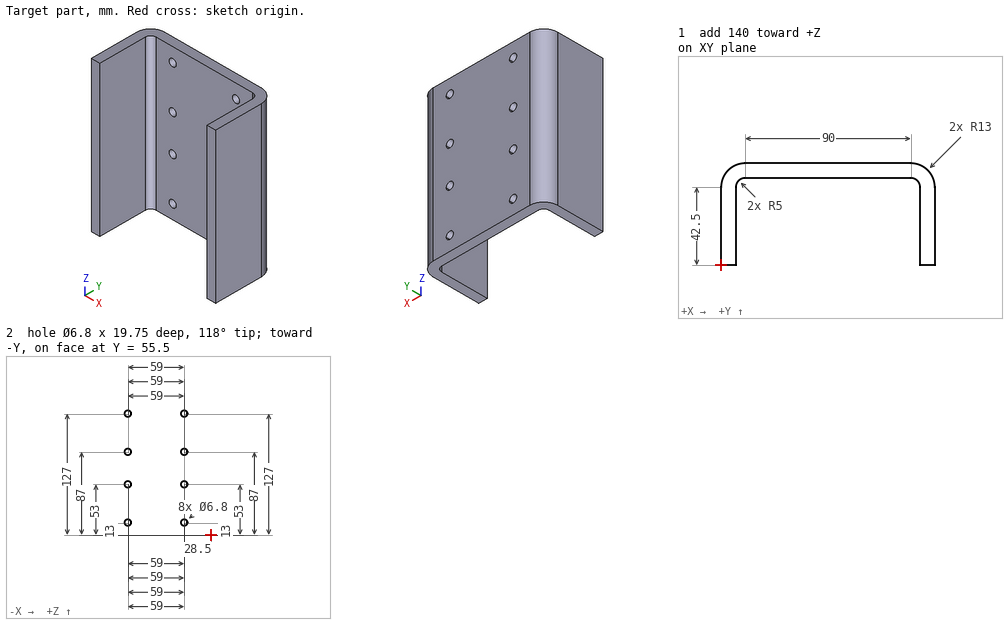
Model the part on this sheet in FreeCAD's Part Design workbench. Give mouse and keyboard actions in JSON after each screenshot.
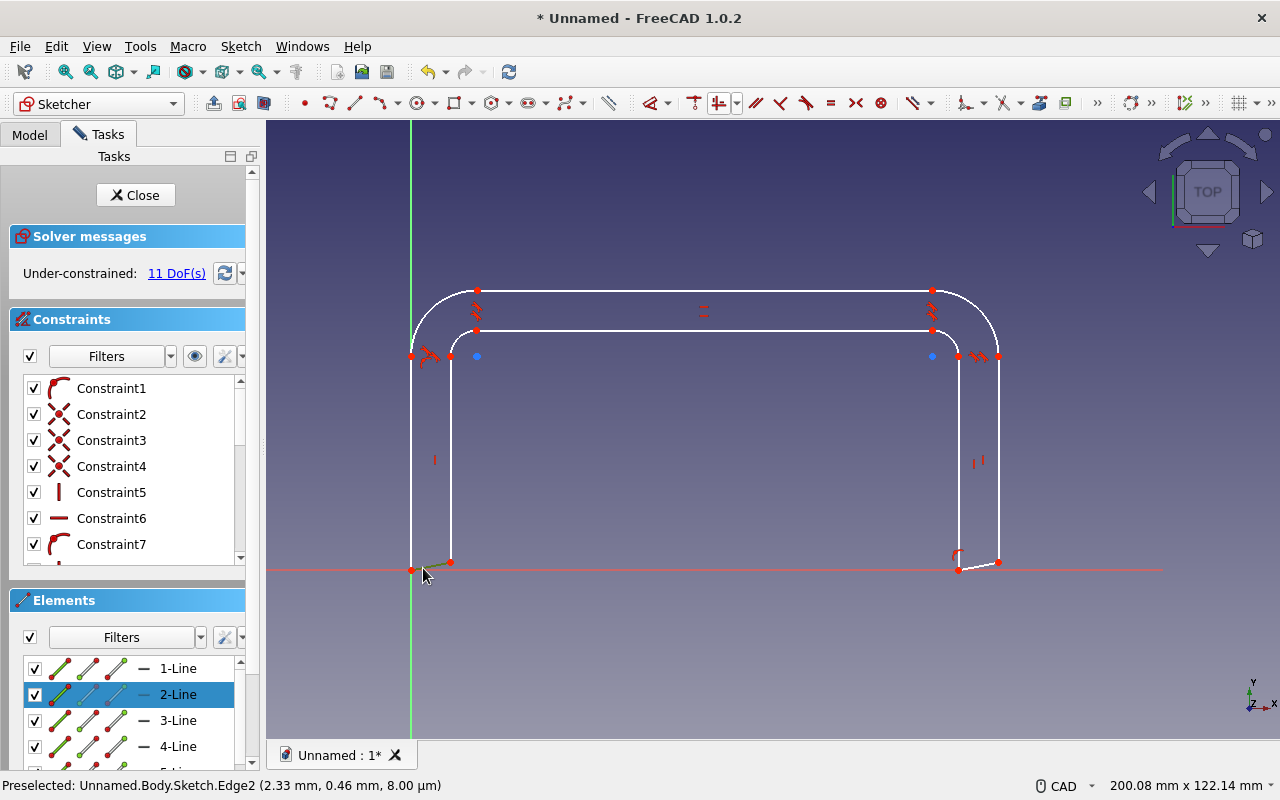
{"action": "key", "text": "h"}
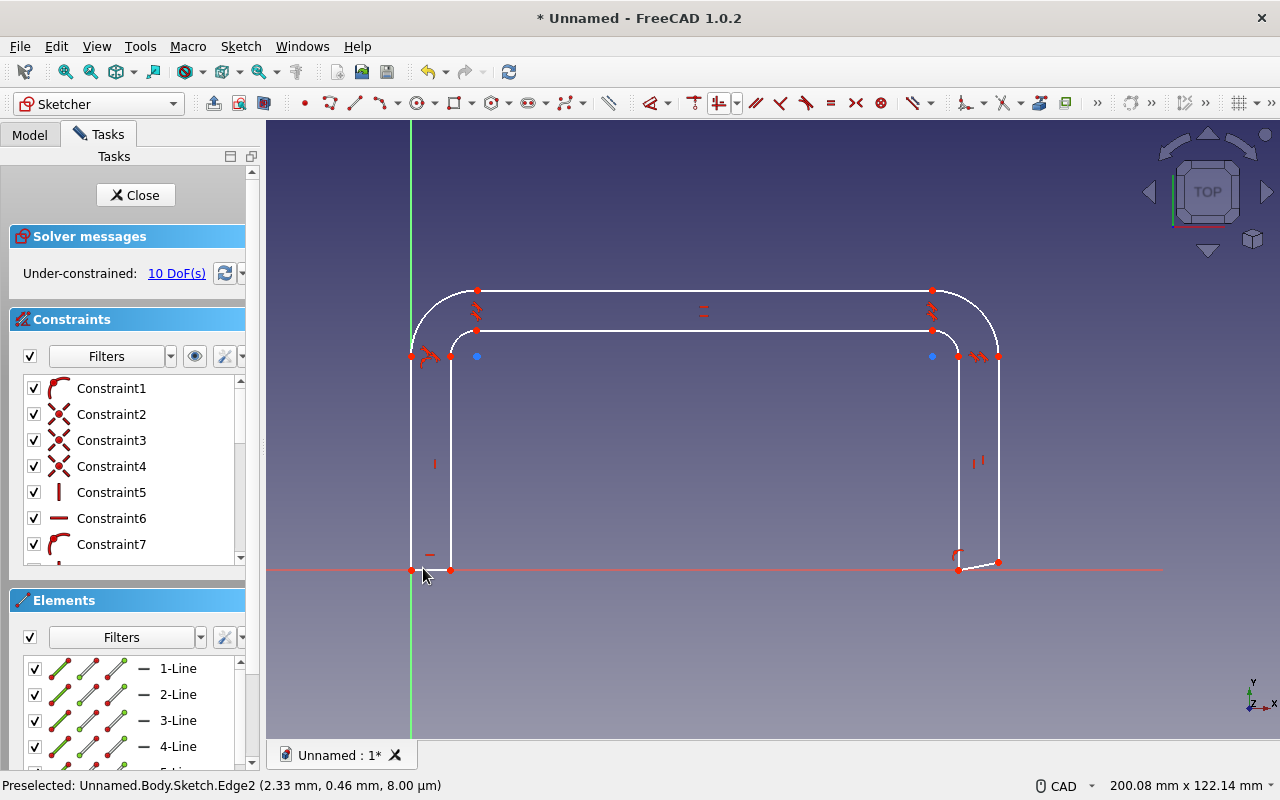
{"action": "left_click", "coordinate": [971, 568]}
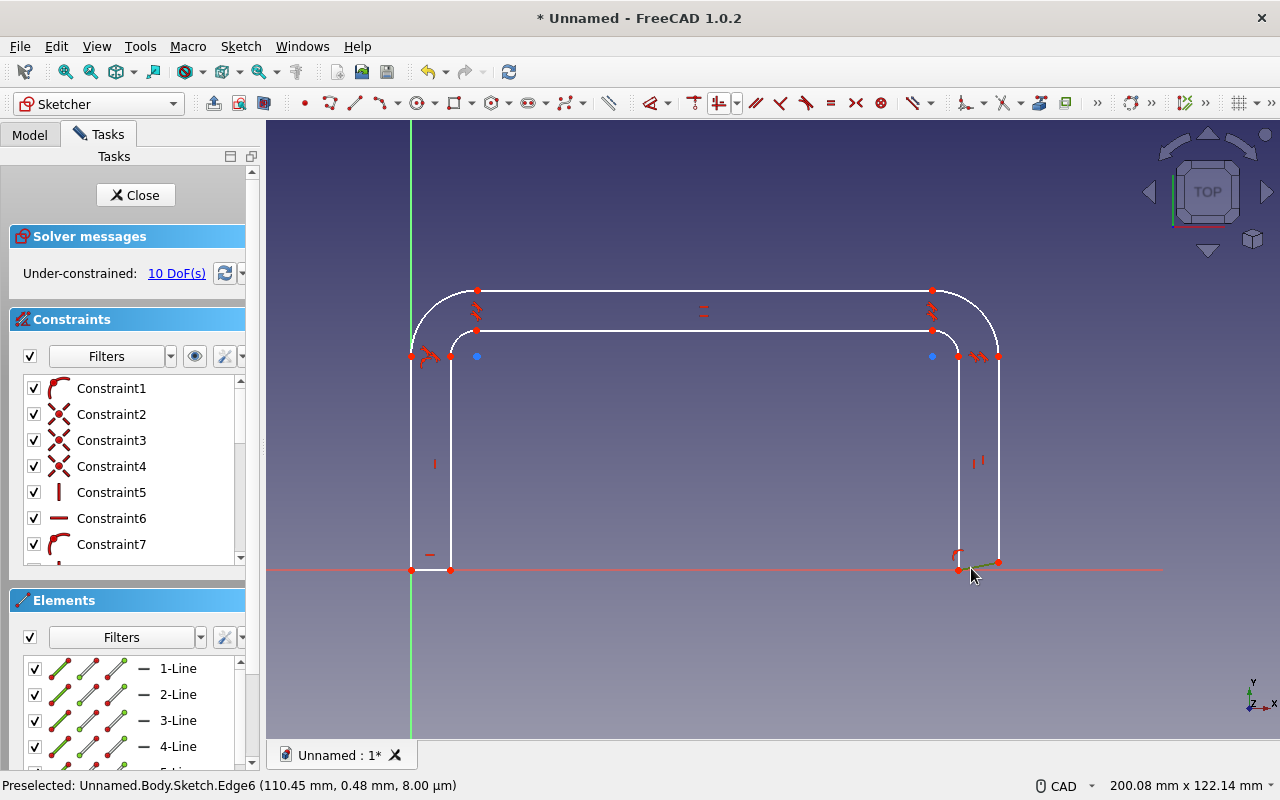
{"action": "left_click", "coordinate": [736, 104]}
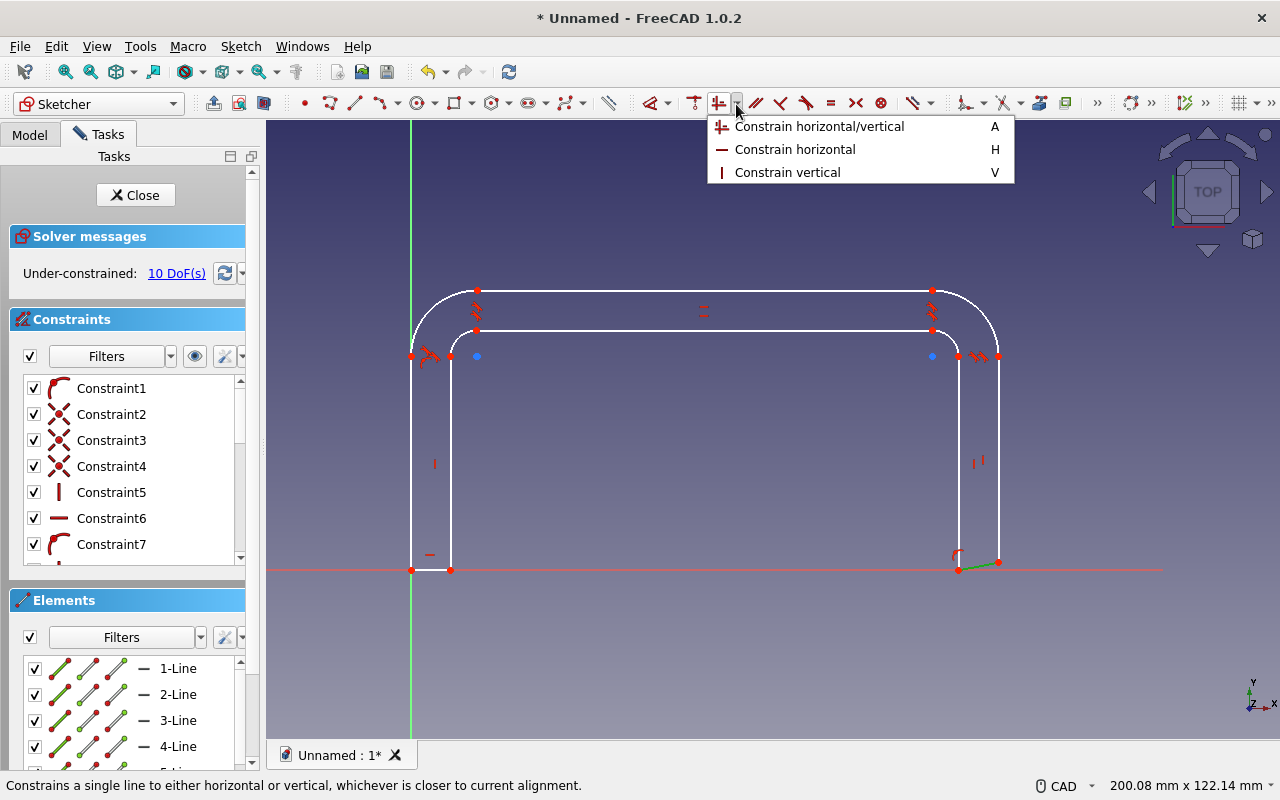
{"action": "left_click", "coordinate": [861, 150]}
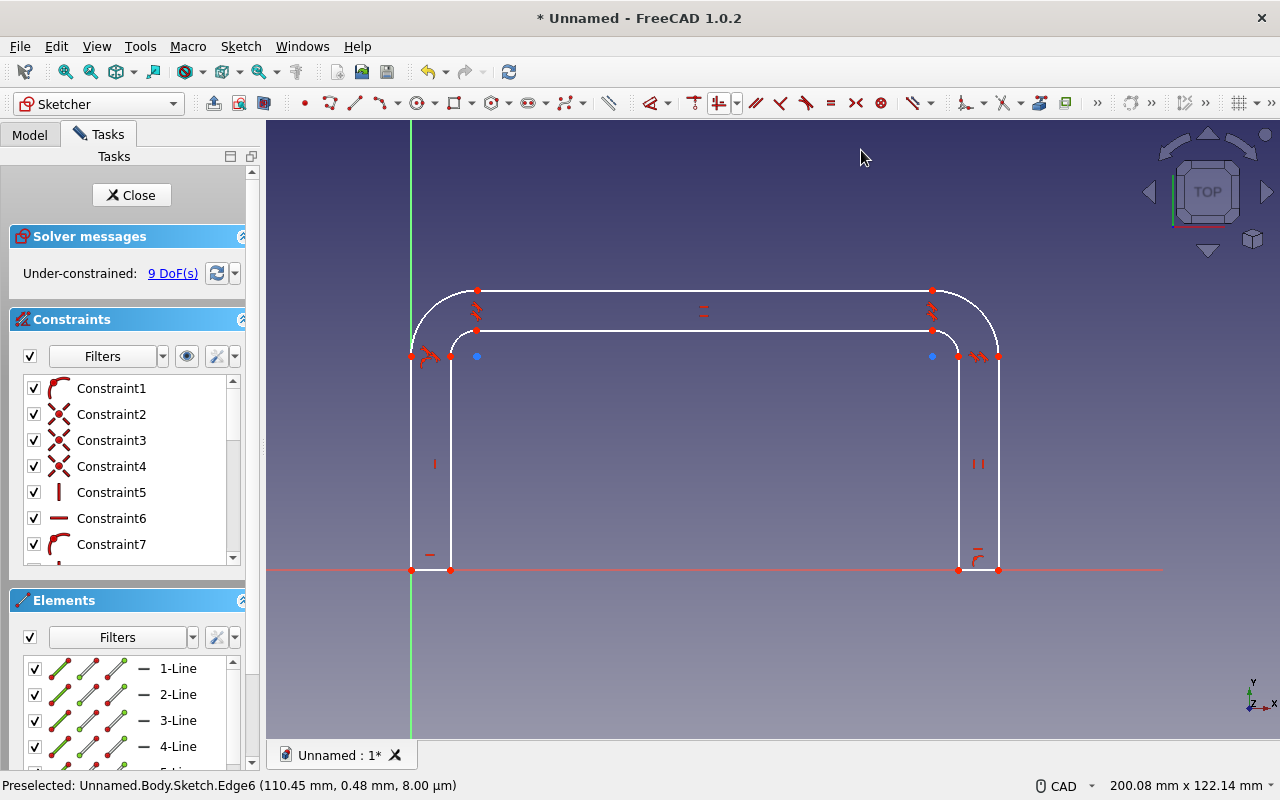
{"action": "left_click", "coordinate": [956, 345]}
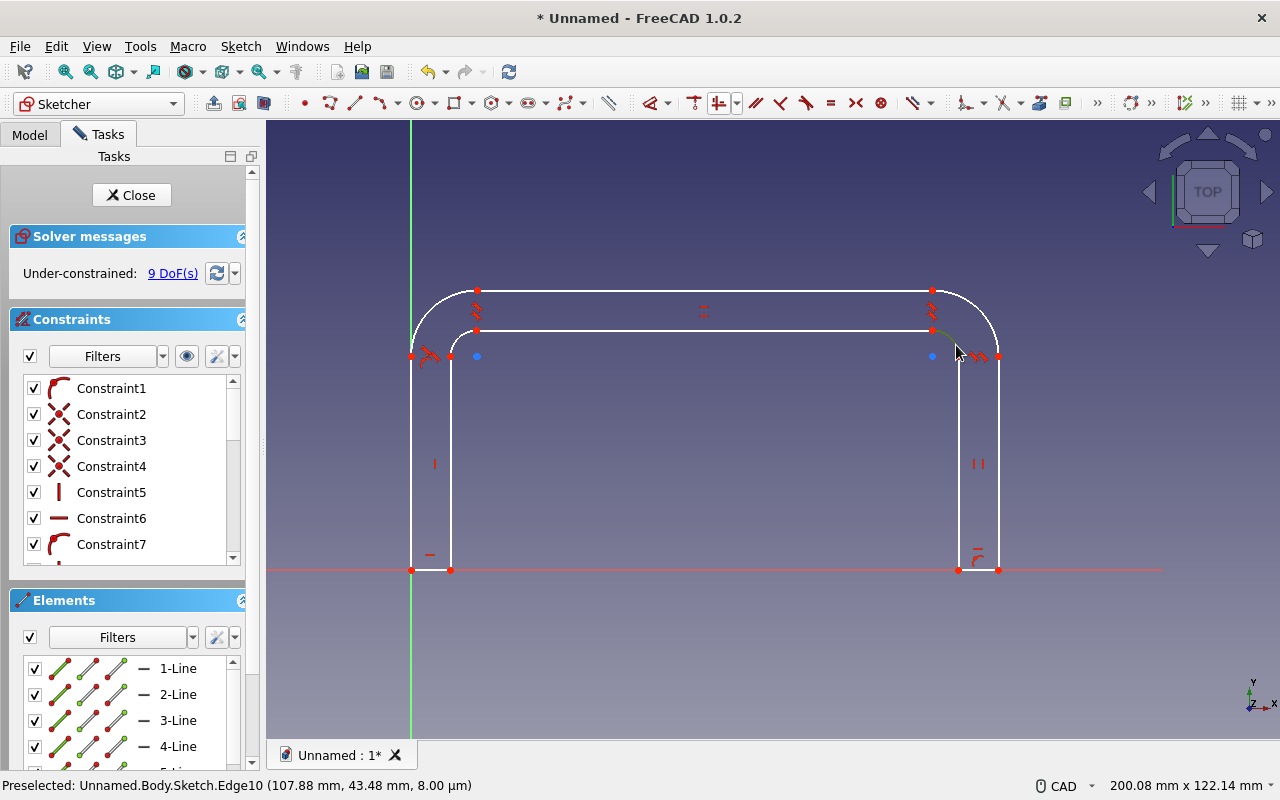
{"action": "left_click", "coordinate": [991, 327]}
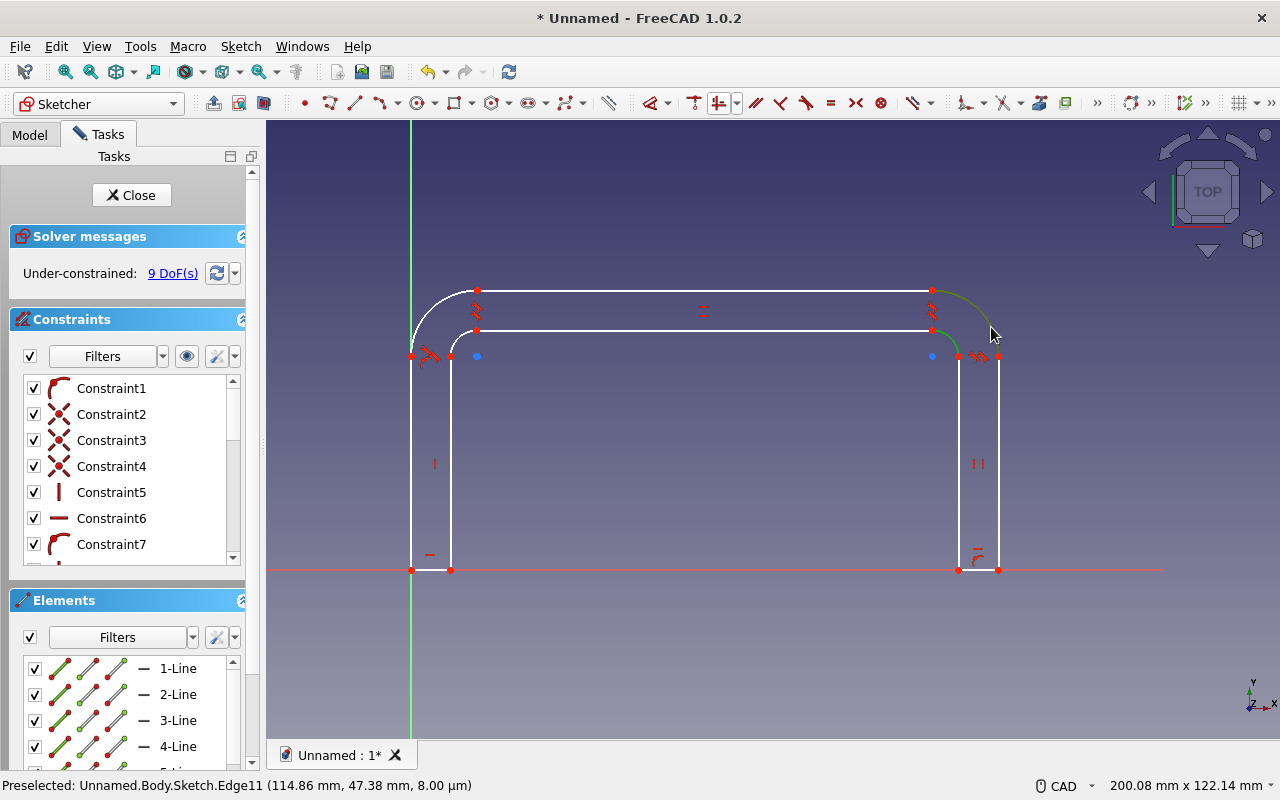
{"action": "key", "text": "c"}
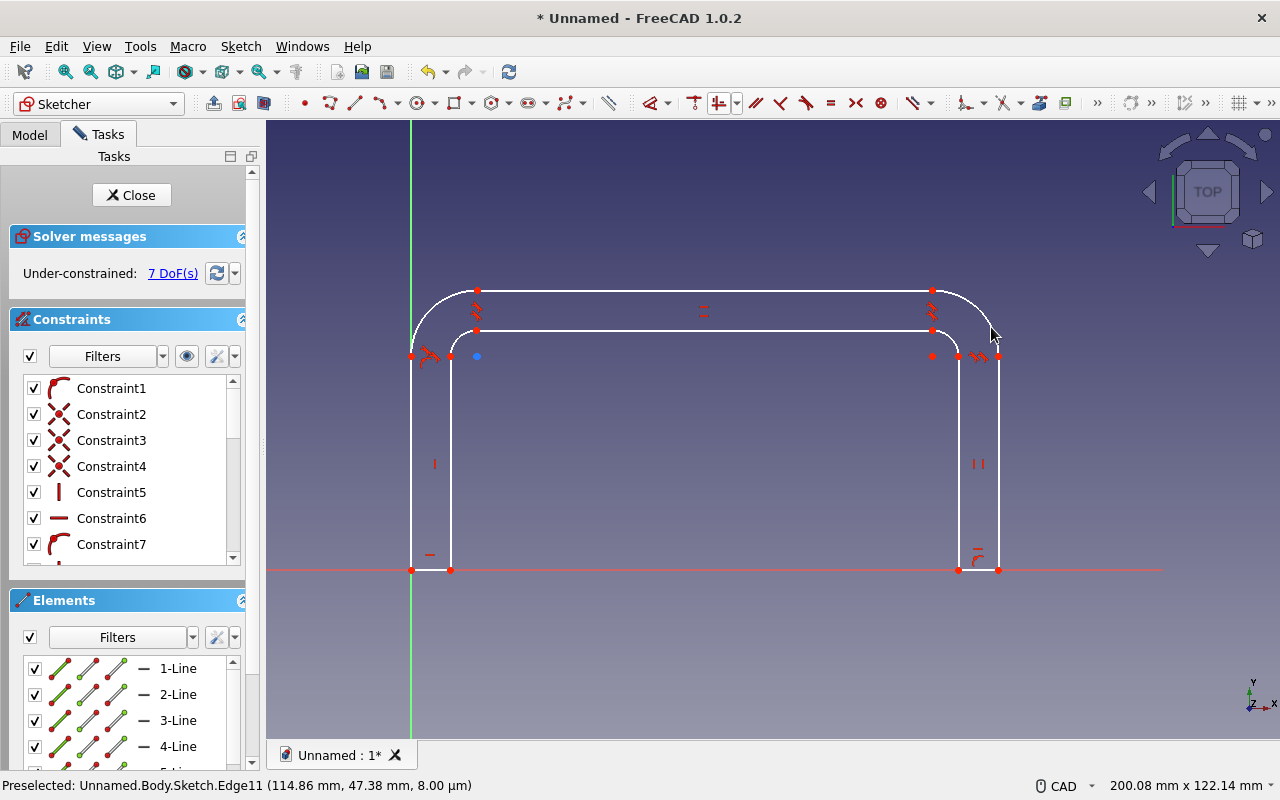
{"action": "left_click", "coordinate": [465, 333]}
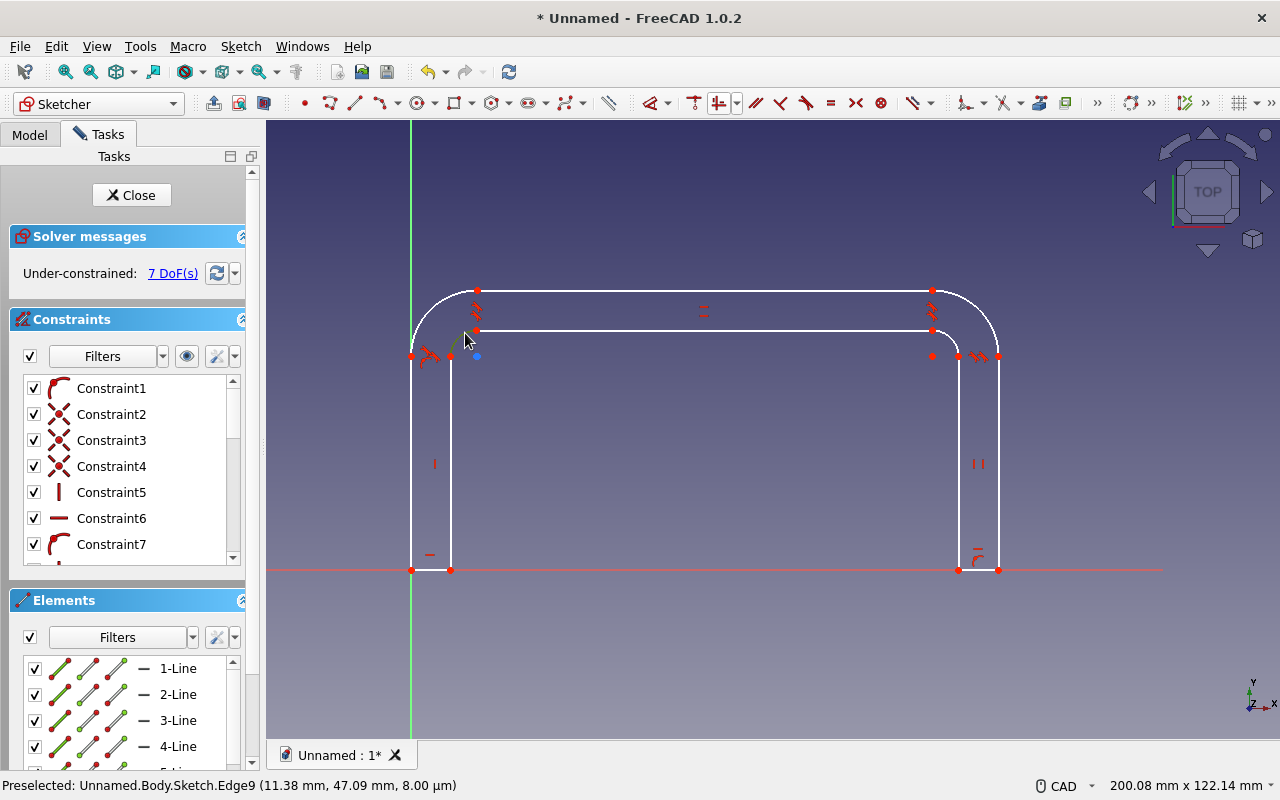
{"action": "left_click", "coordinate": [447, 298]}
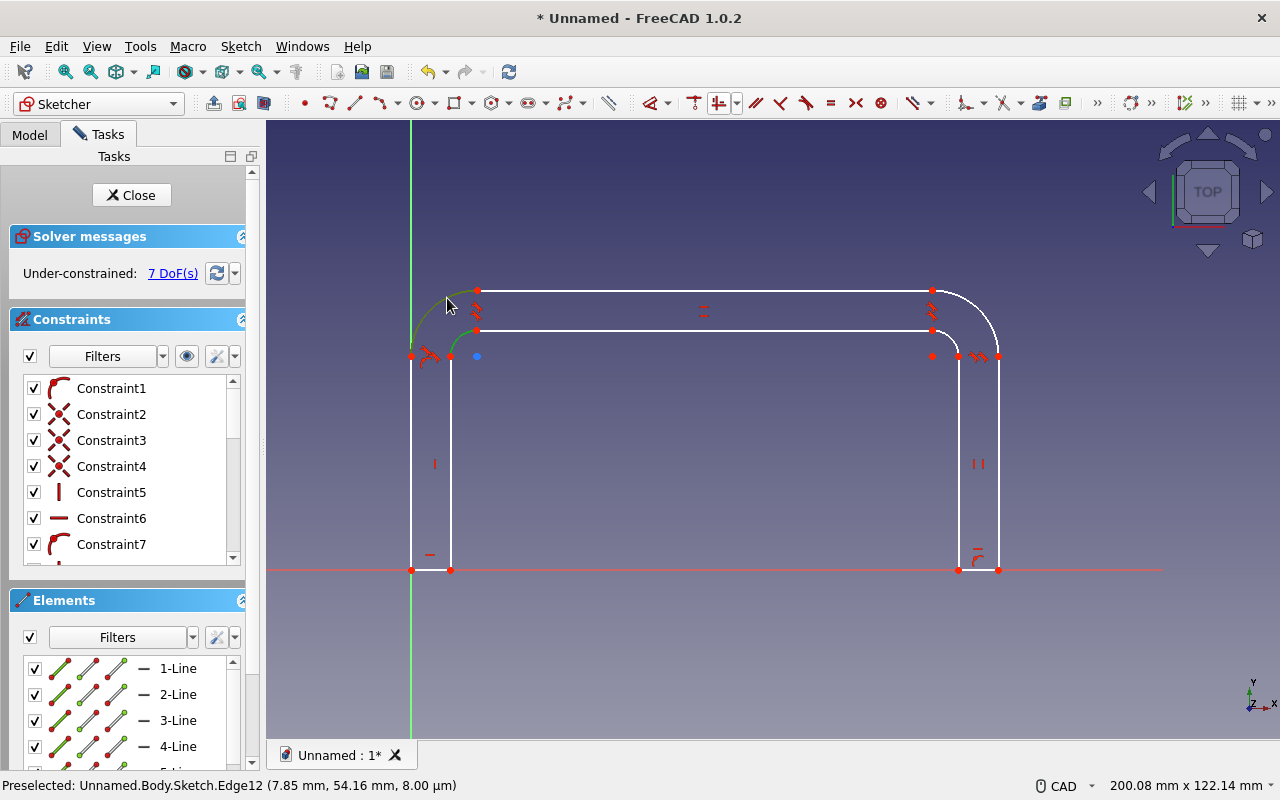
{"action": "key", "text": "c"}